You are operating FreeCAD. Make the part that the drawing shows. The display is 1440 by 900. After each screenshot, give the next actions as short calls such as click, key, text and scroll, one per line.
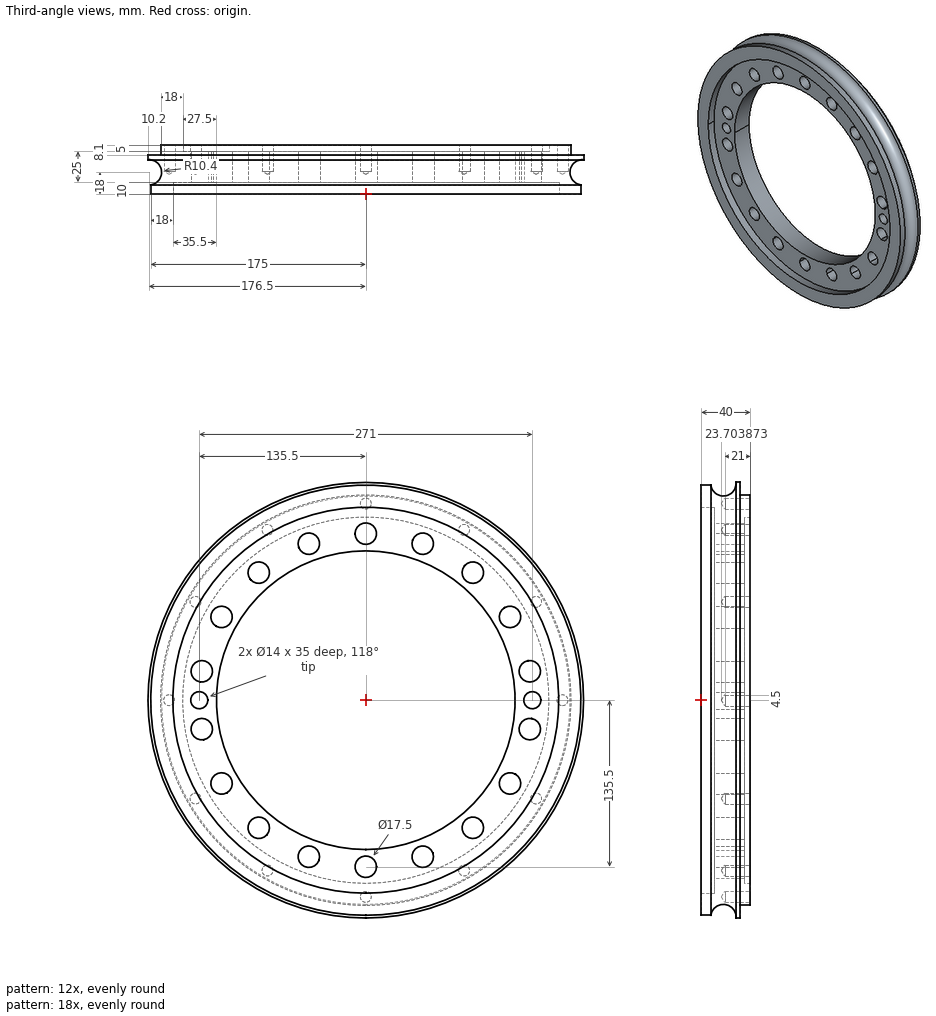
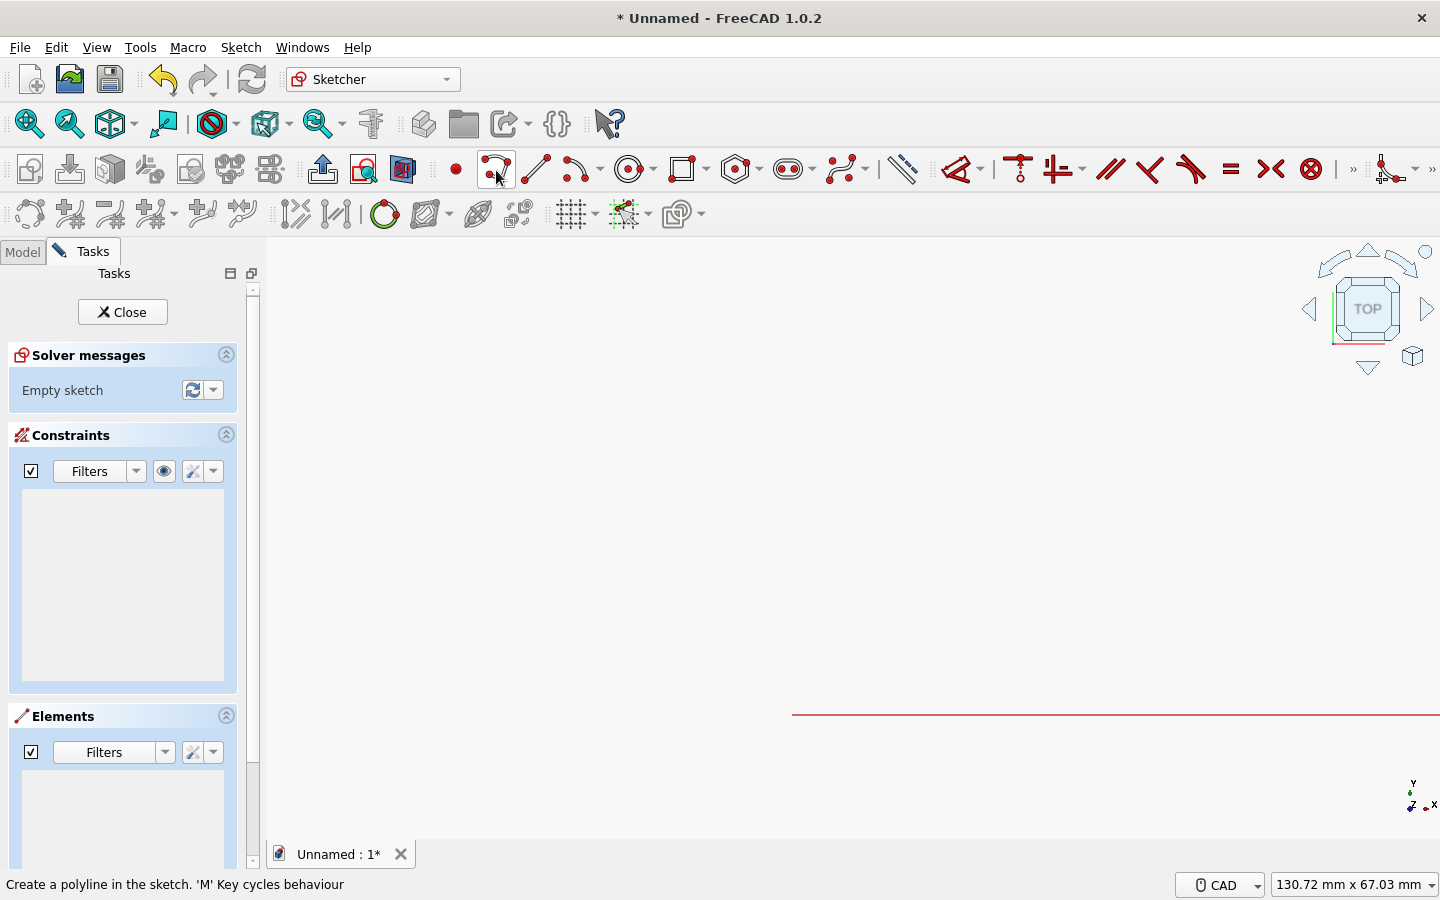
click(553, 646)
click(553, 715)
click(715, 706)
click(715, 625)
click(1034, 625)
click(1034, 401)
click(787, 401)
click(787, 356)
click(625, 356)
click(625, 429)
click(534, 429)
click(534, 460)
right_click(534, 460)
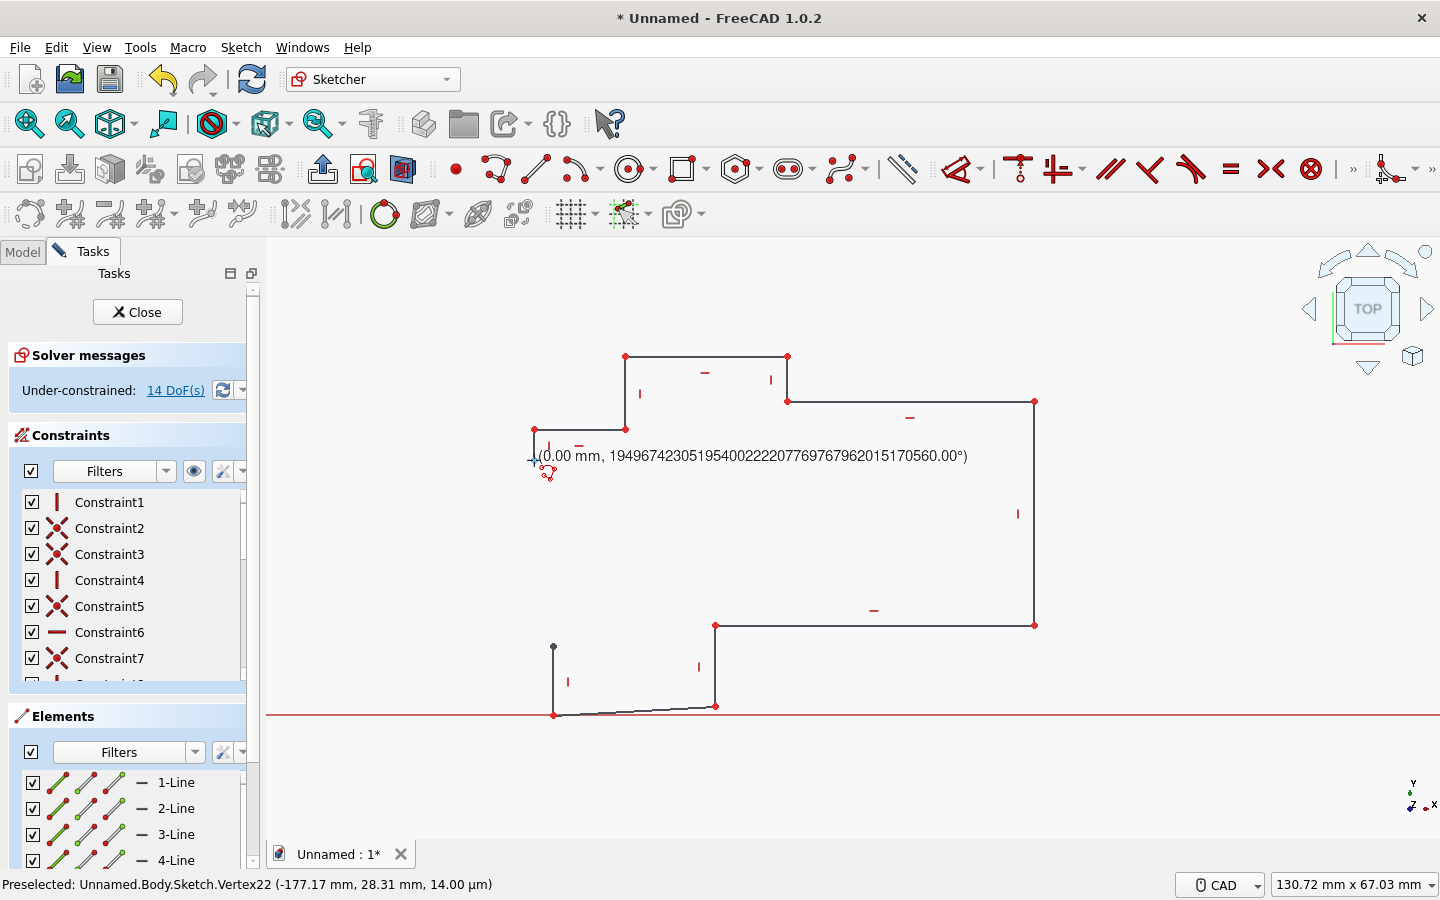
key(g)
key(3)
key(a)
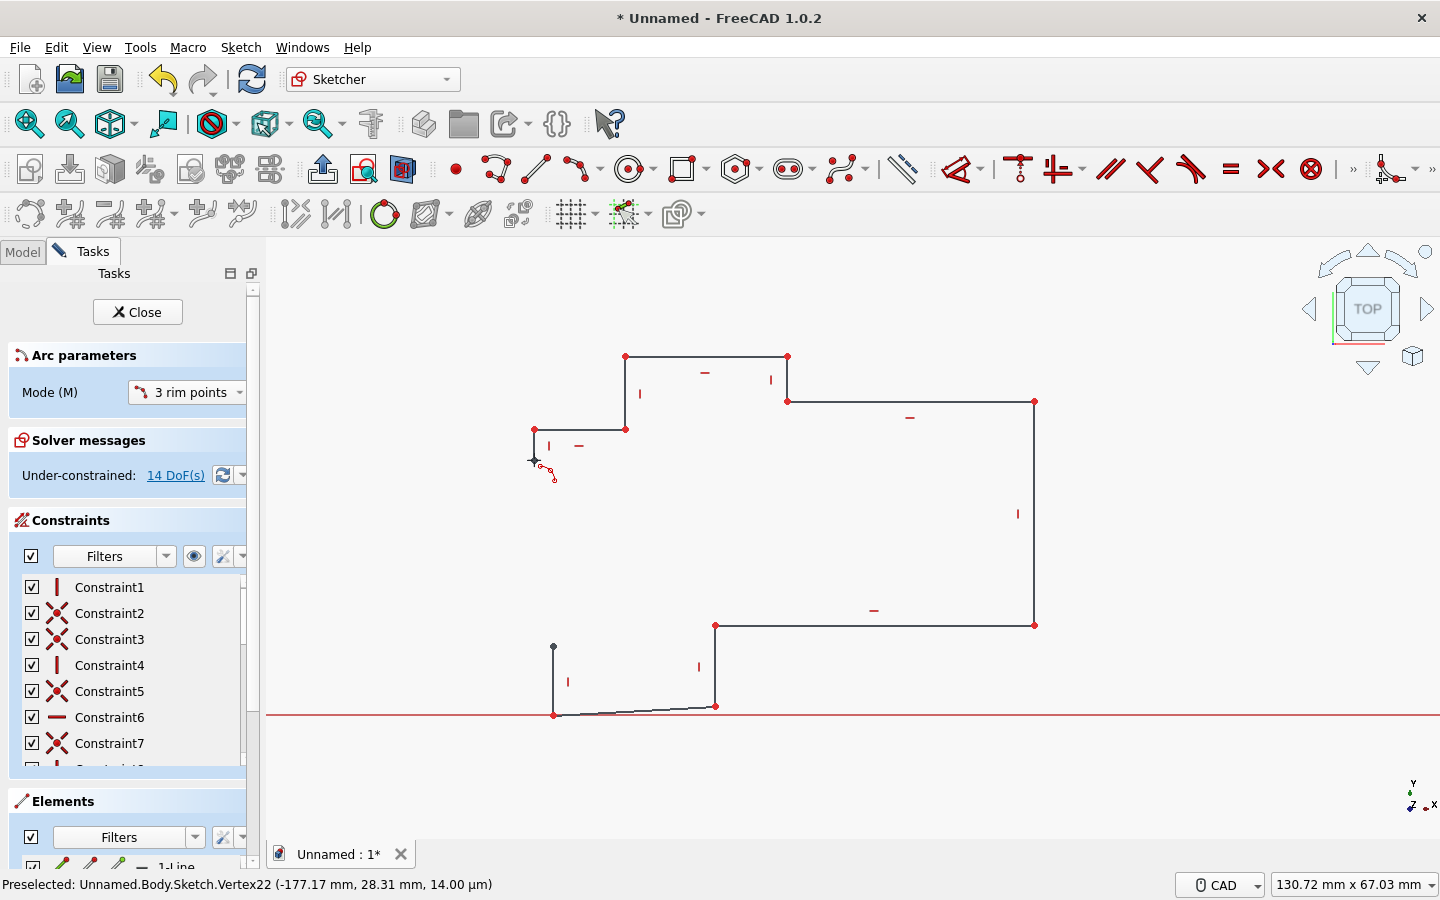
click(534, 461)
click(553, 647)
click(633, 544)
key(Escape)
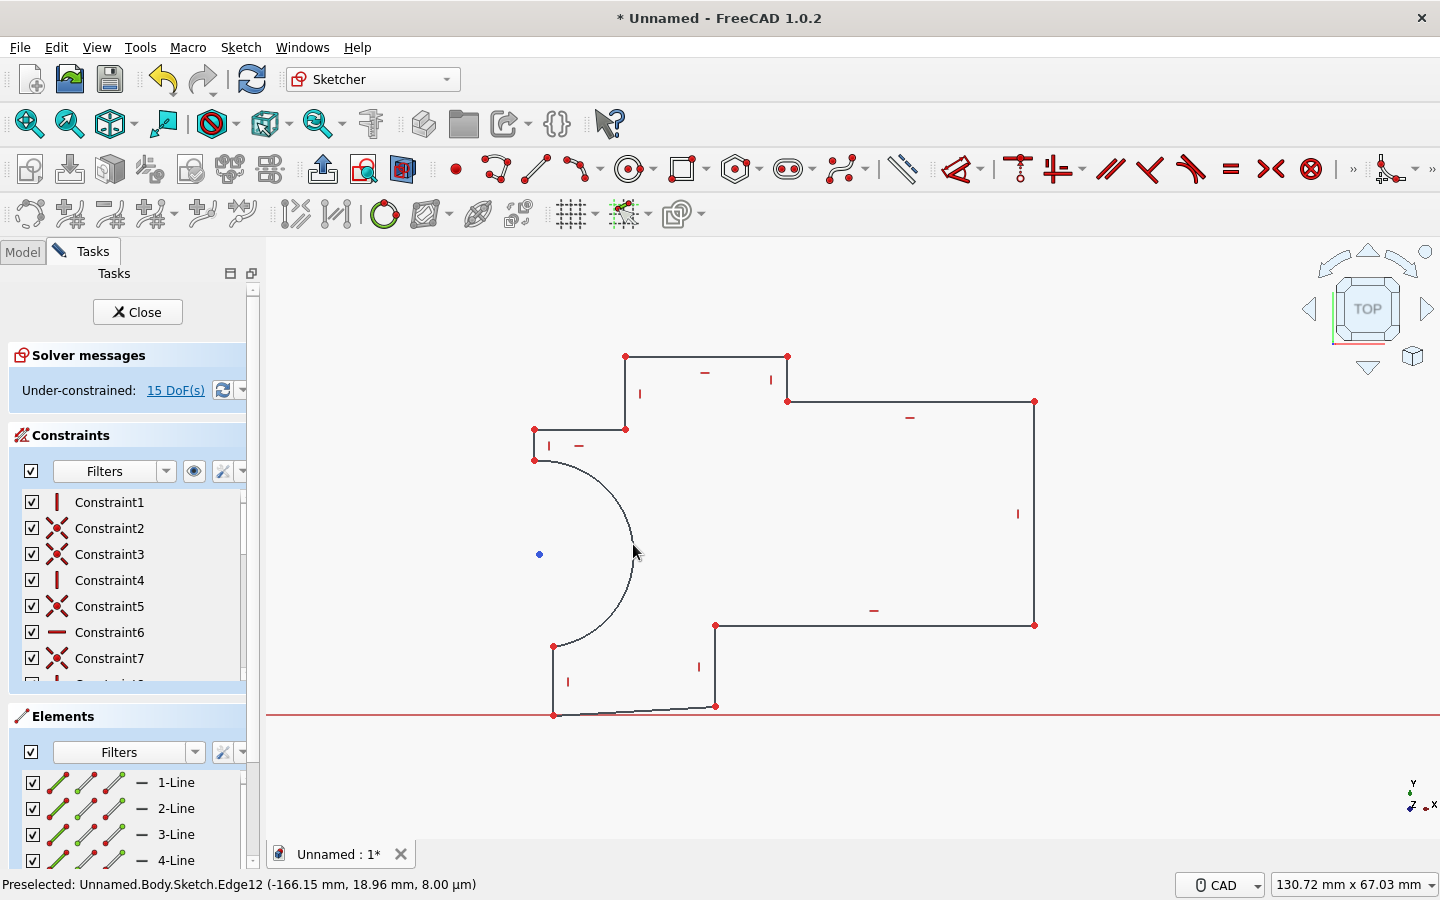
click(602, 713)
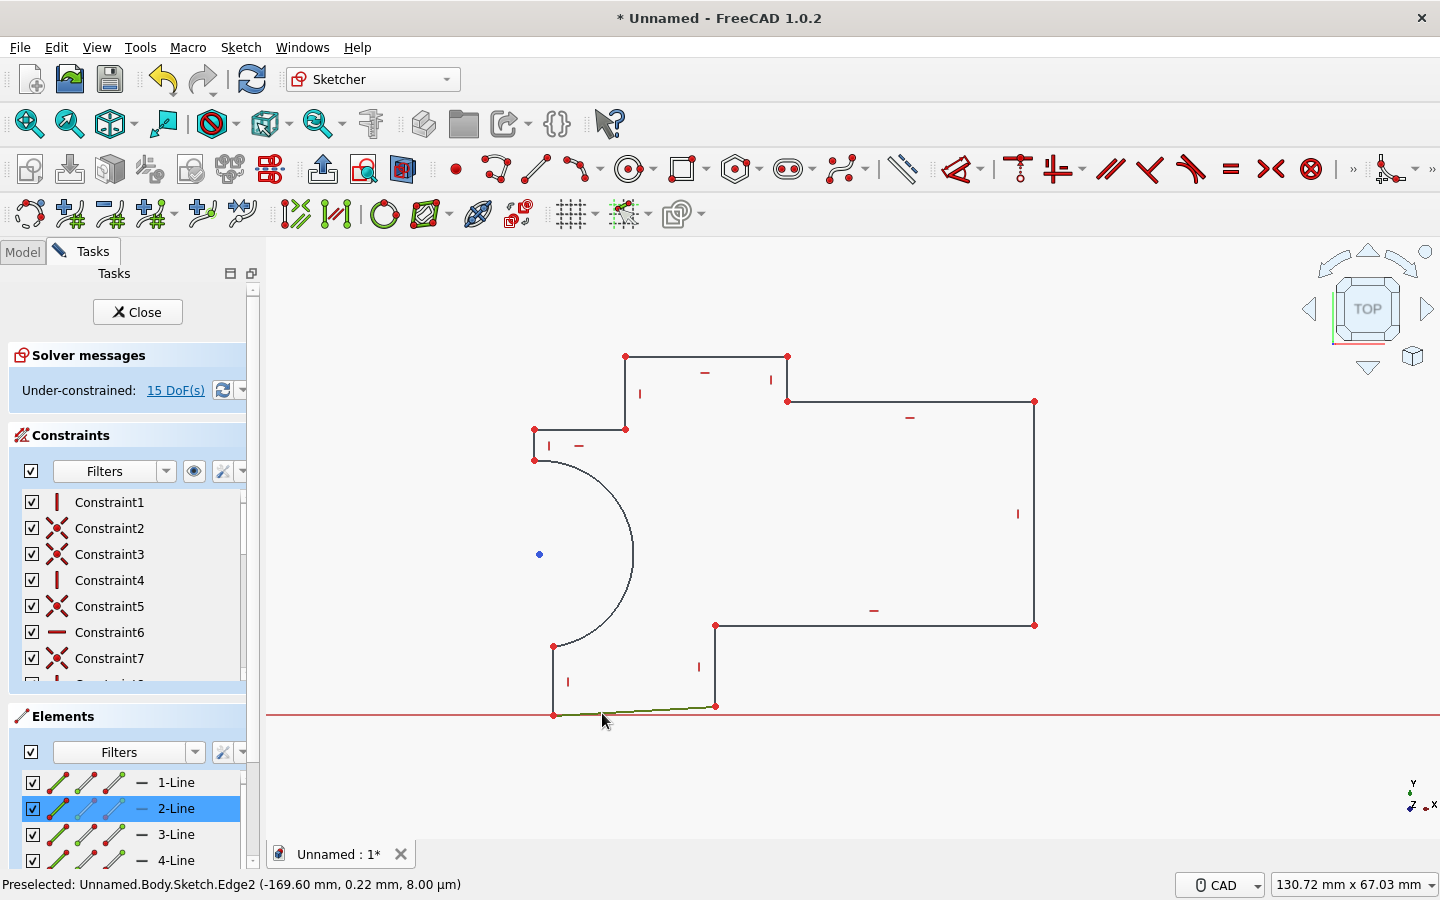
key(h)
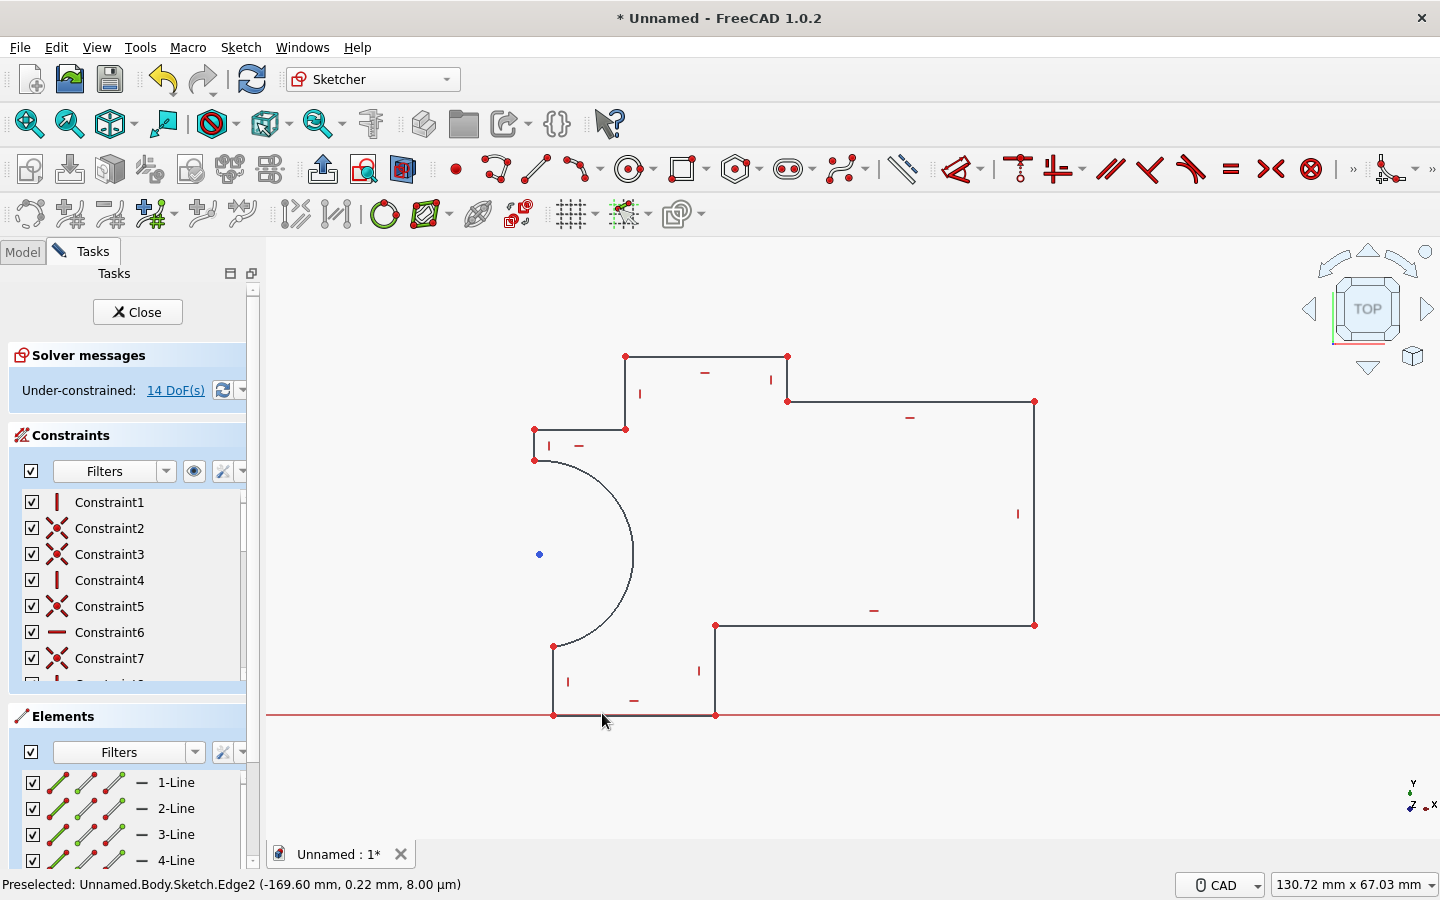
click(956, 170)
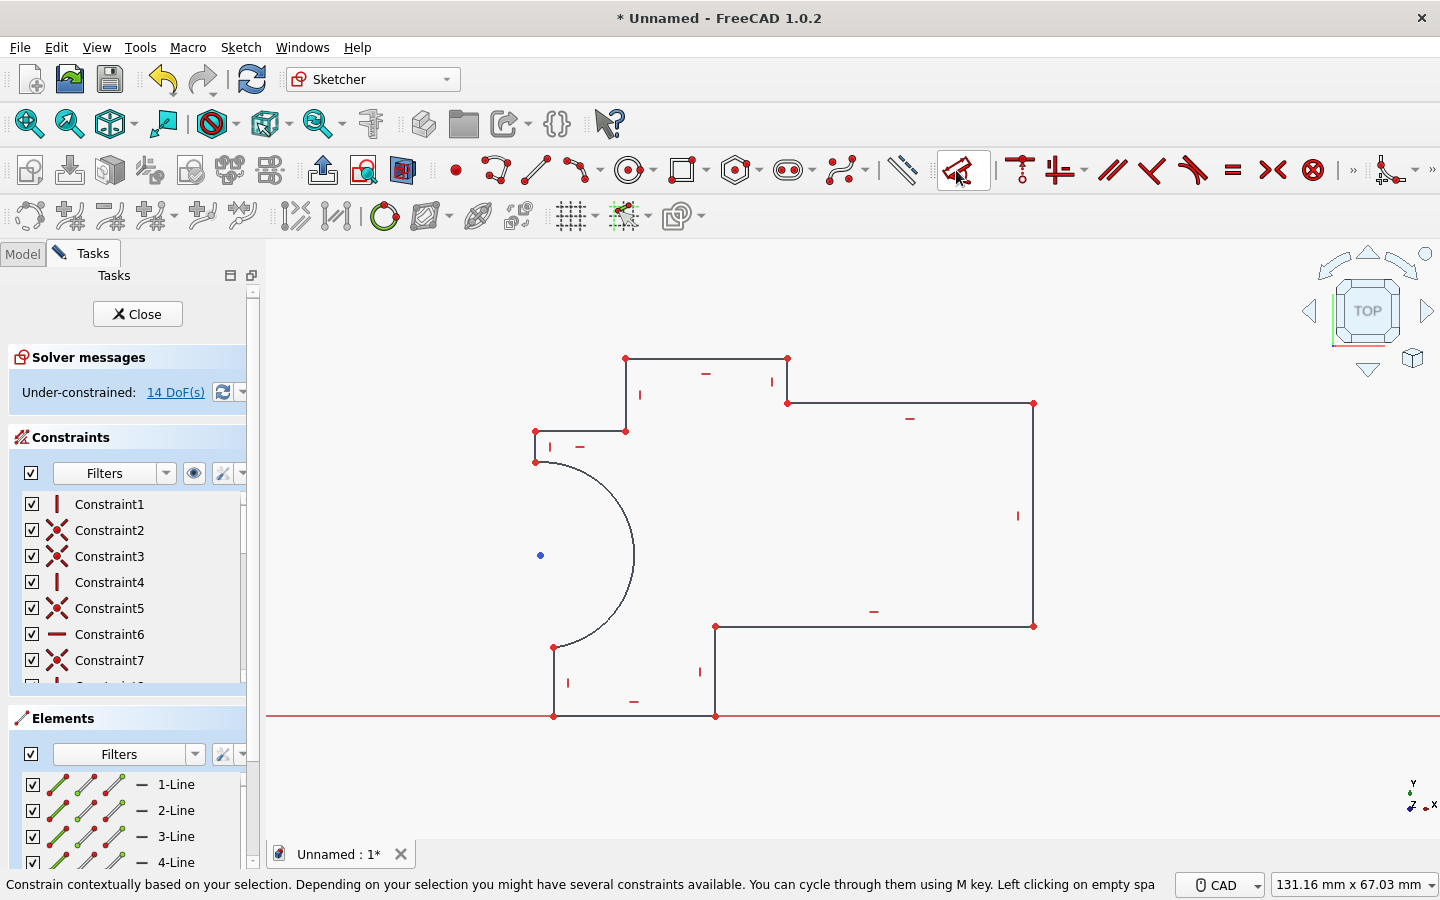
click(622, 601)
click(650, 617)